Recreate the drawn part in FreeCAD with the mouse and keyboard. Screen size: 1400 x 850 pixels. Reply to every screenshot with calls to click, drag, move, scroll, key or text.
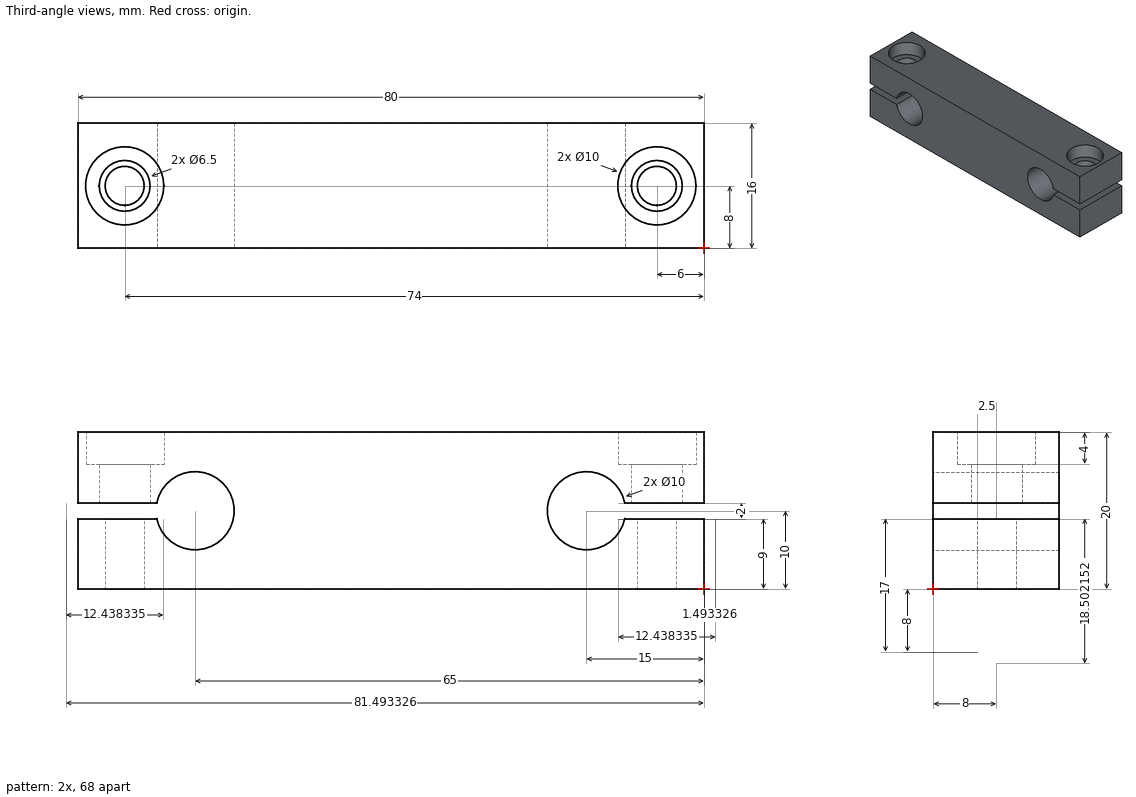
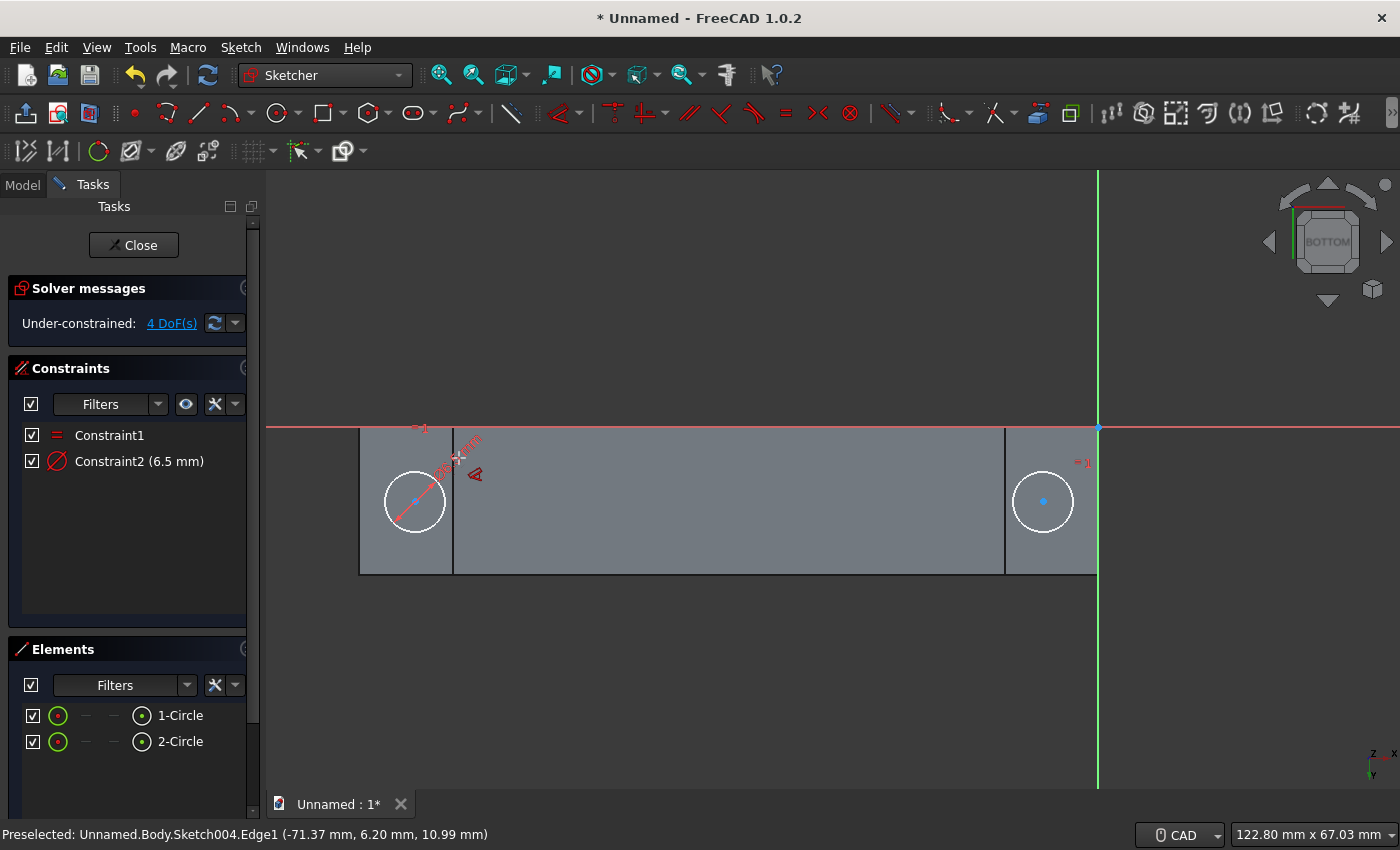
click(415, 502)
click(1132, 465)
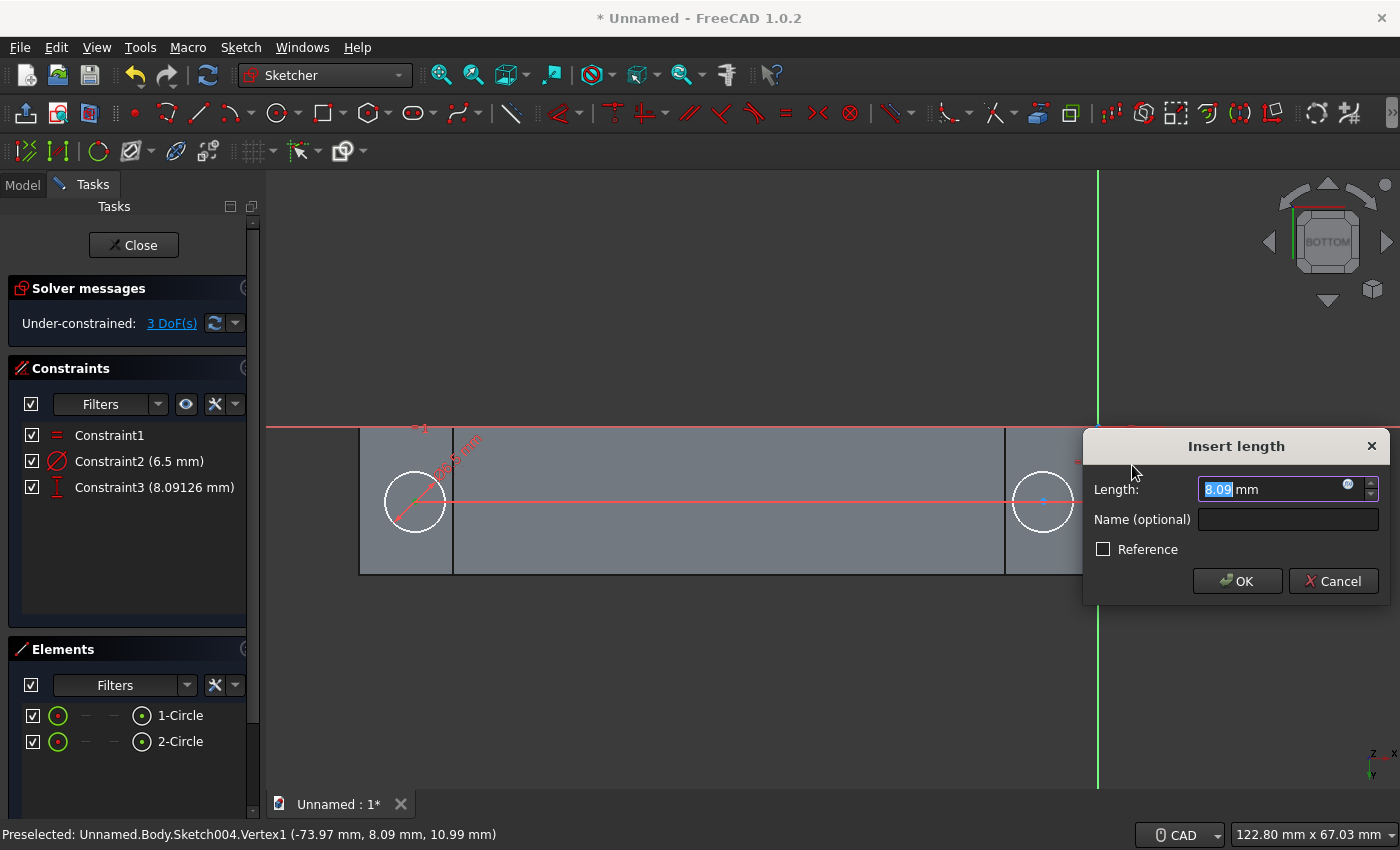
text(8)
key(Return)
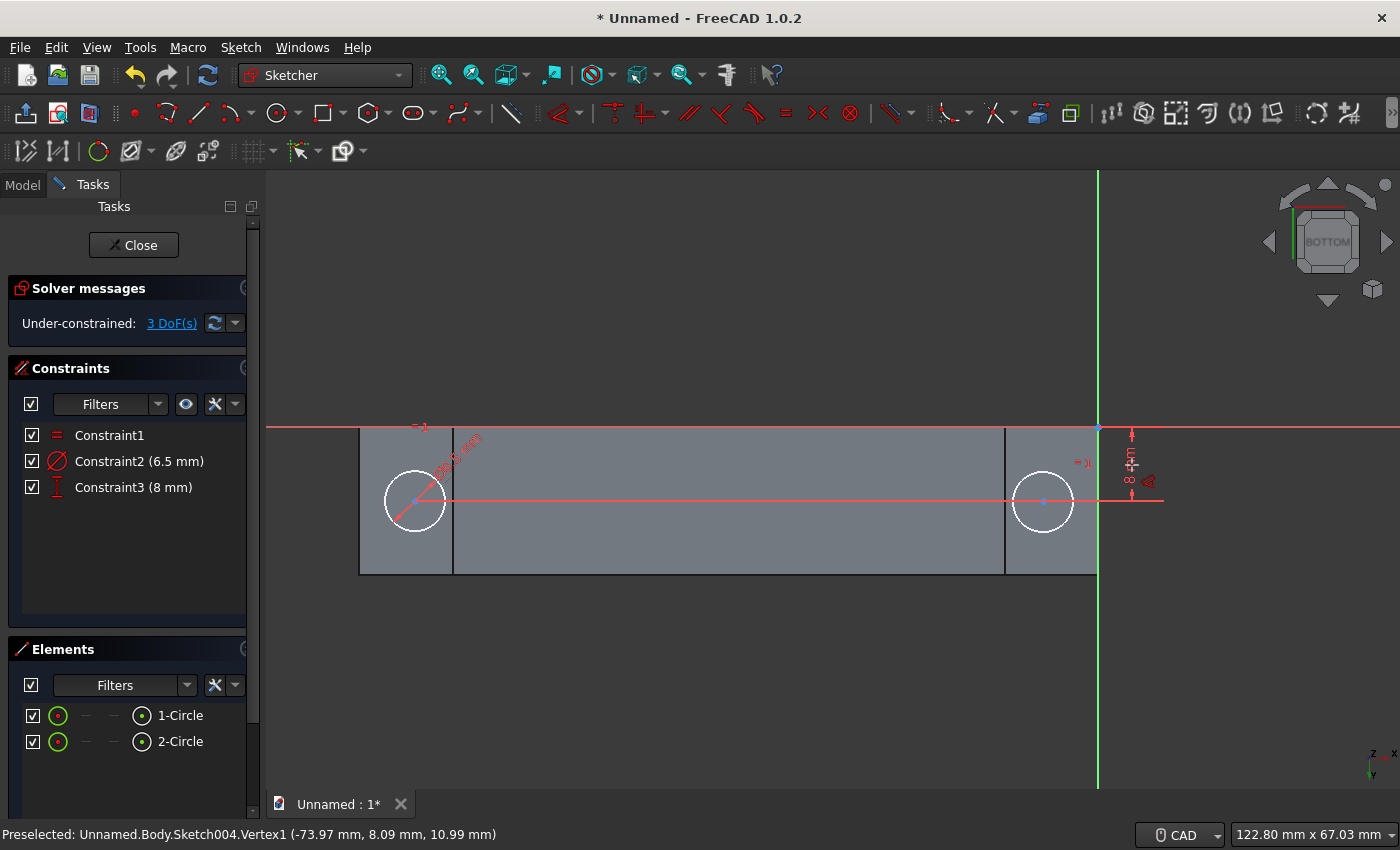
click(1043, 502)
click(1071, 393)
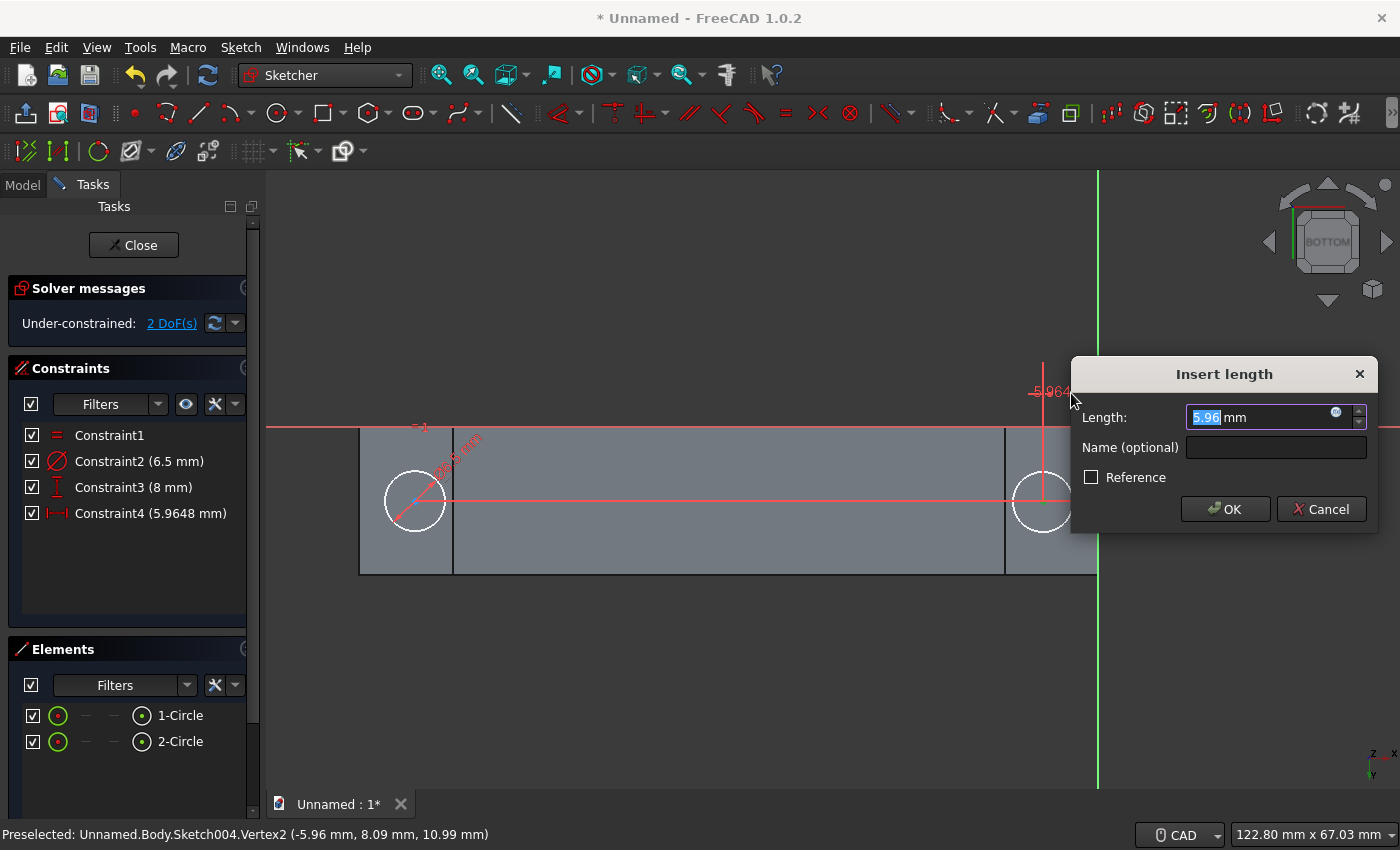
text(6)
key(Return)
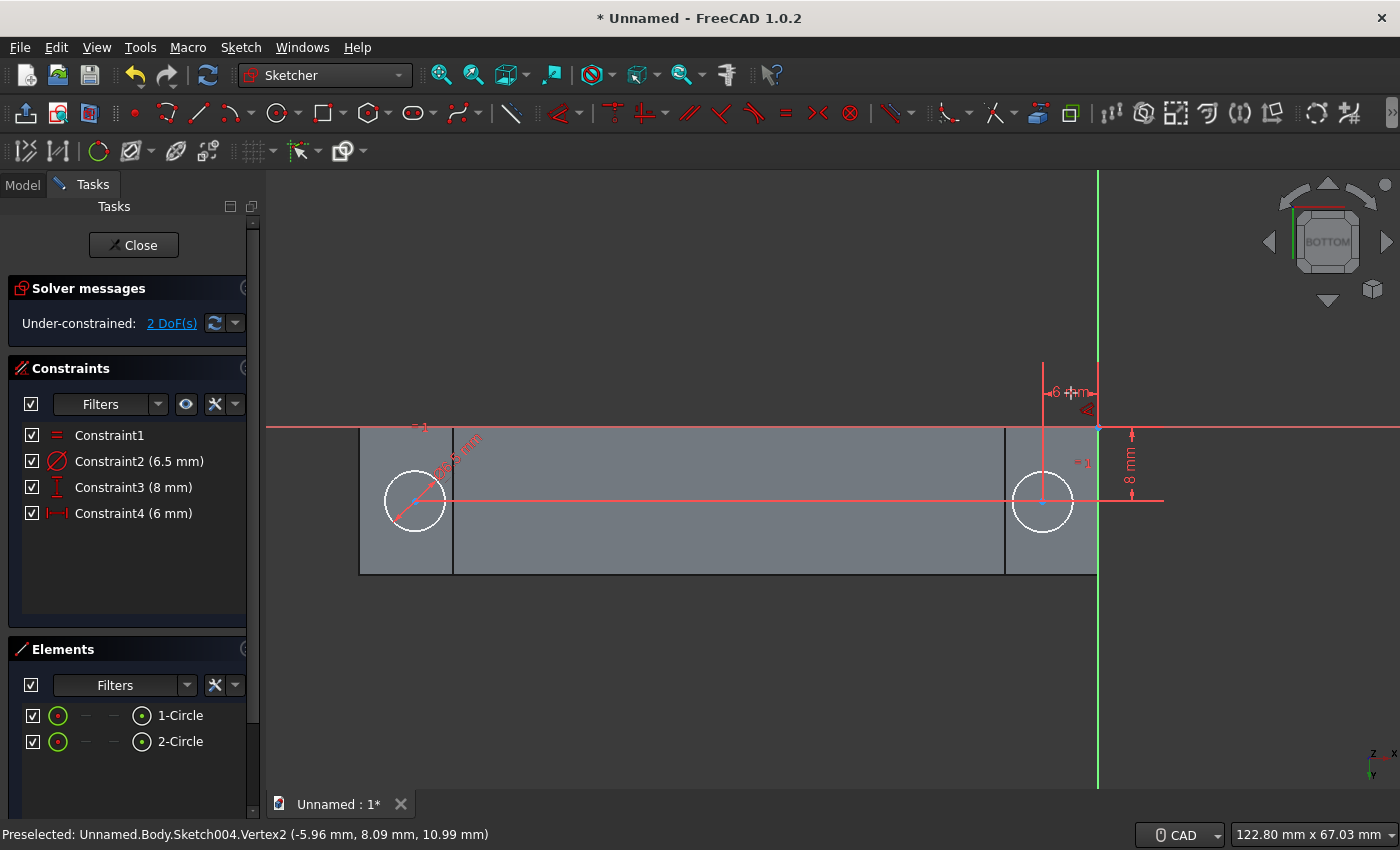
click(1043, 502)
click(1132, 491)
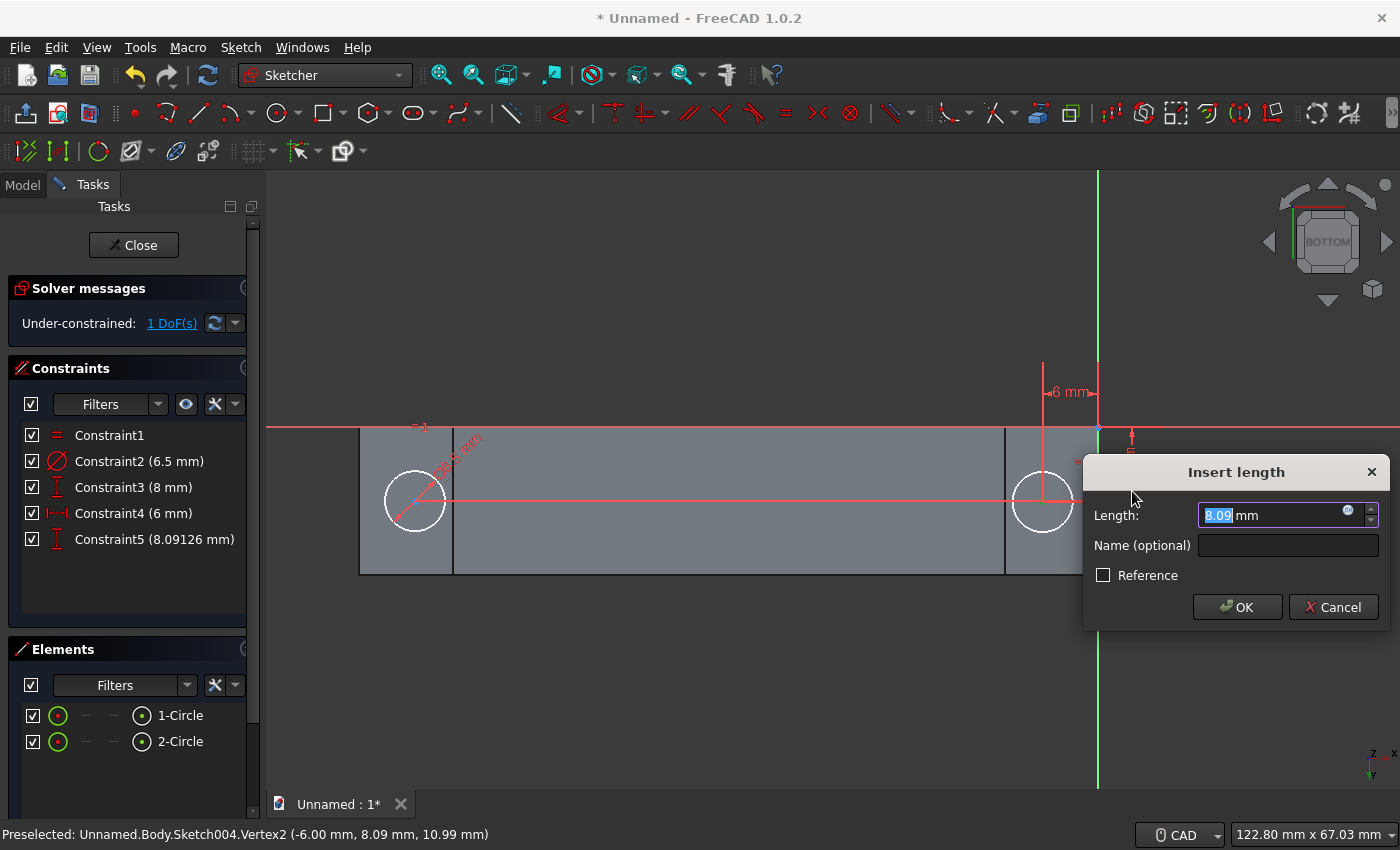
text(8)
key(Return)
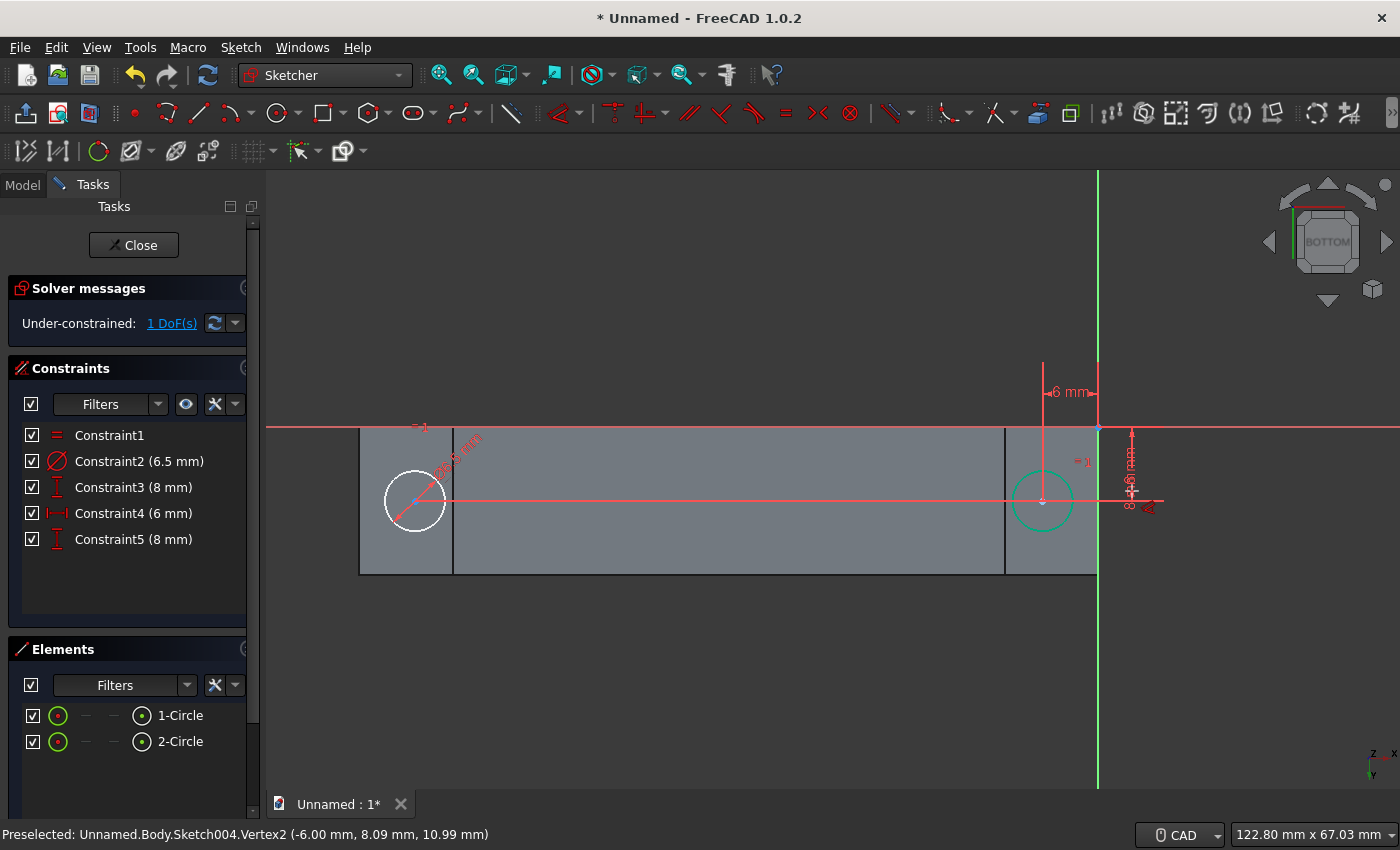
click(415, 501)
click(757, 393)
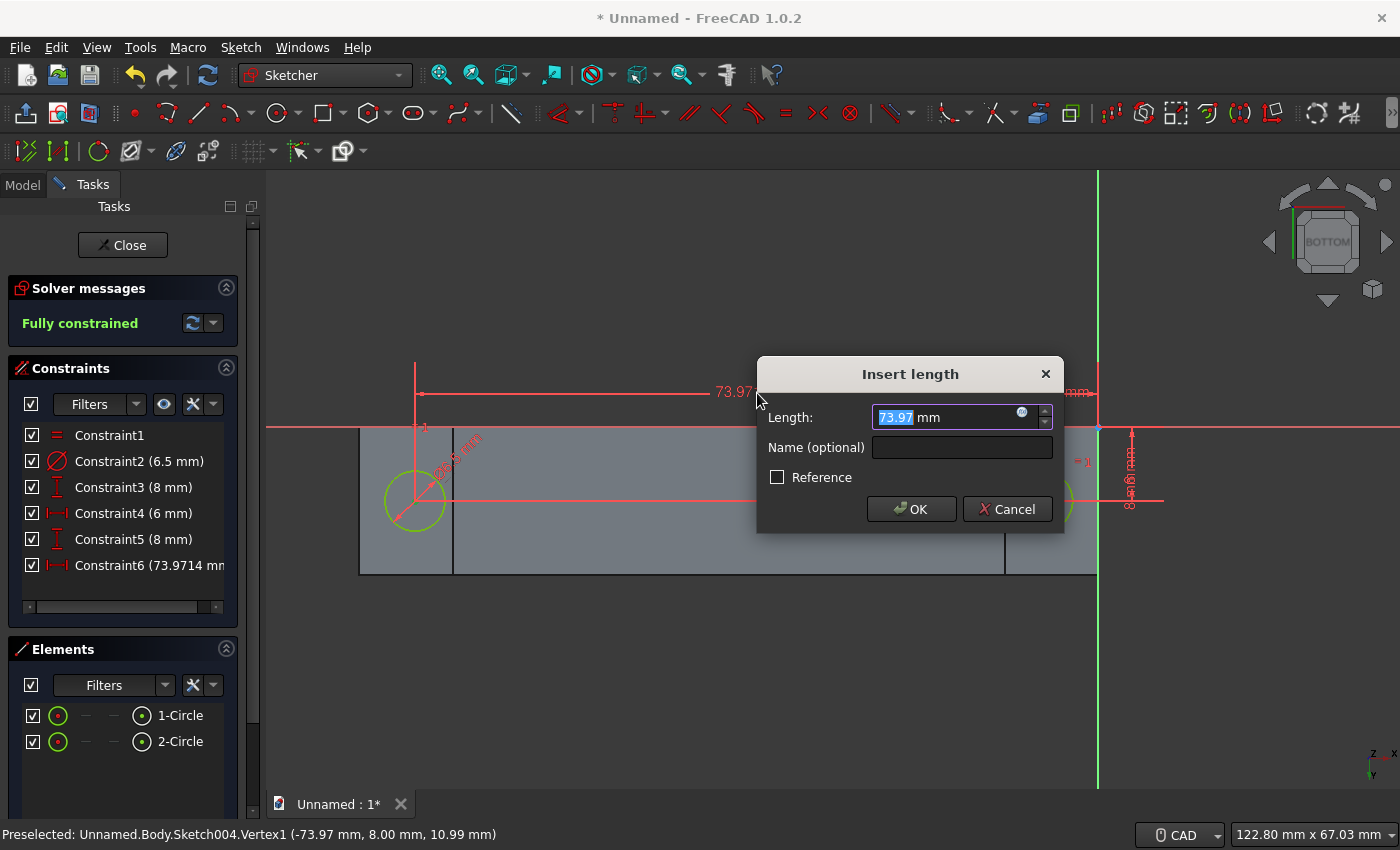
text(74)
key(Return)
key(Escape)